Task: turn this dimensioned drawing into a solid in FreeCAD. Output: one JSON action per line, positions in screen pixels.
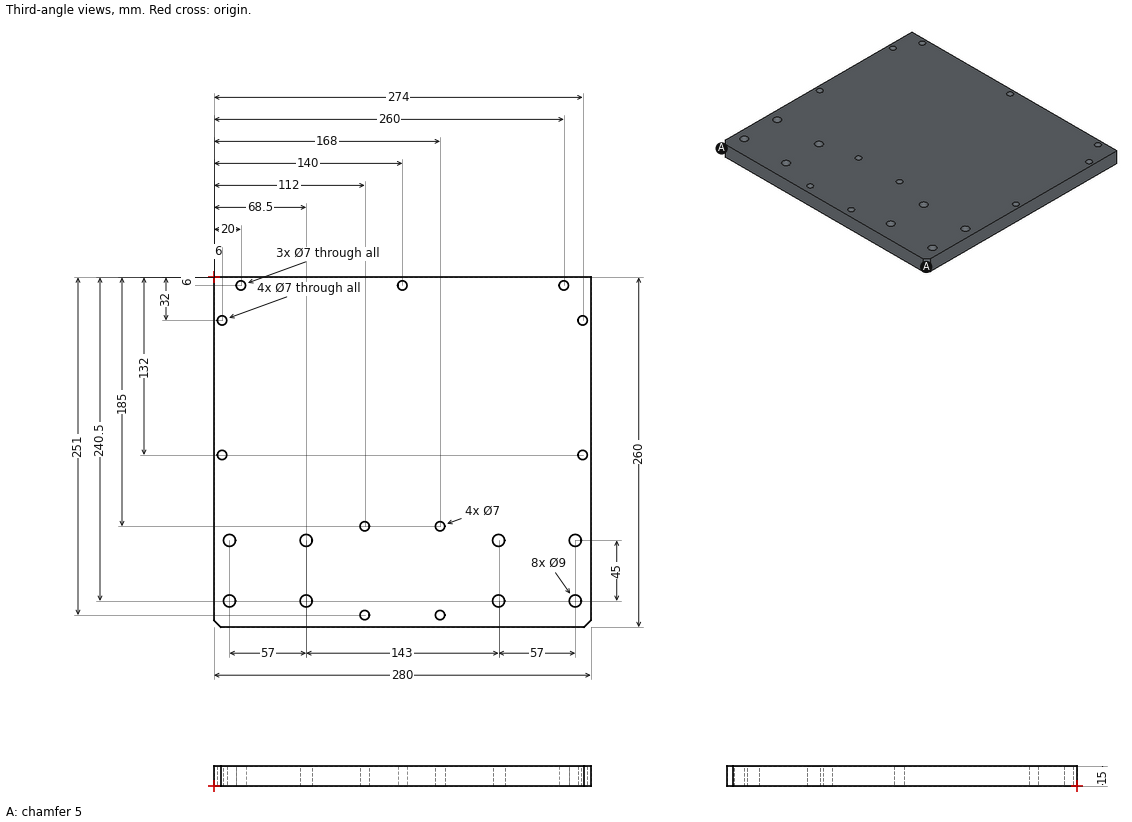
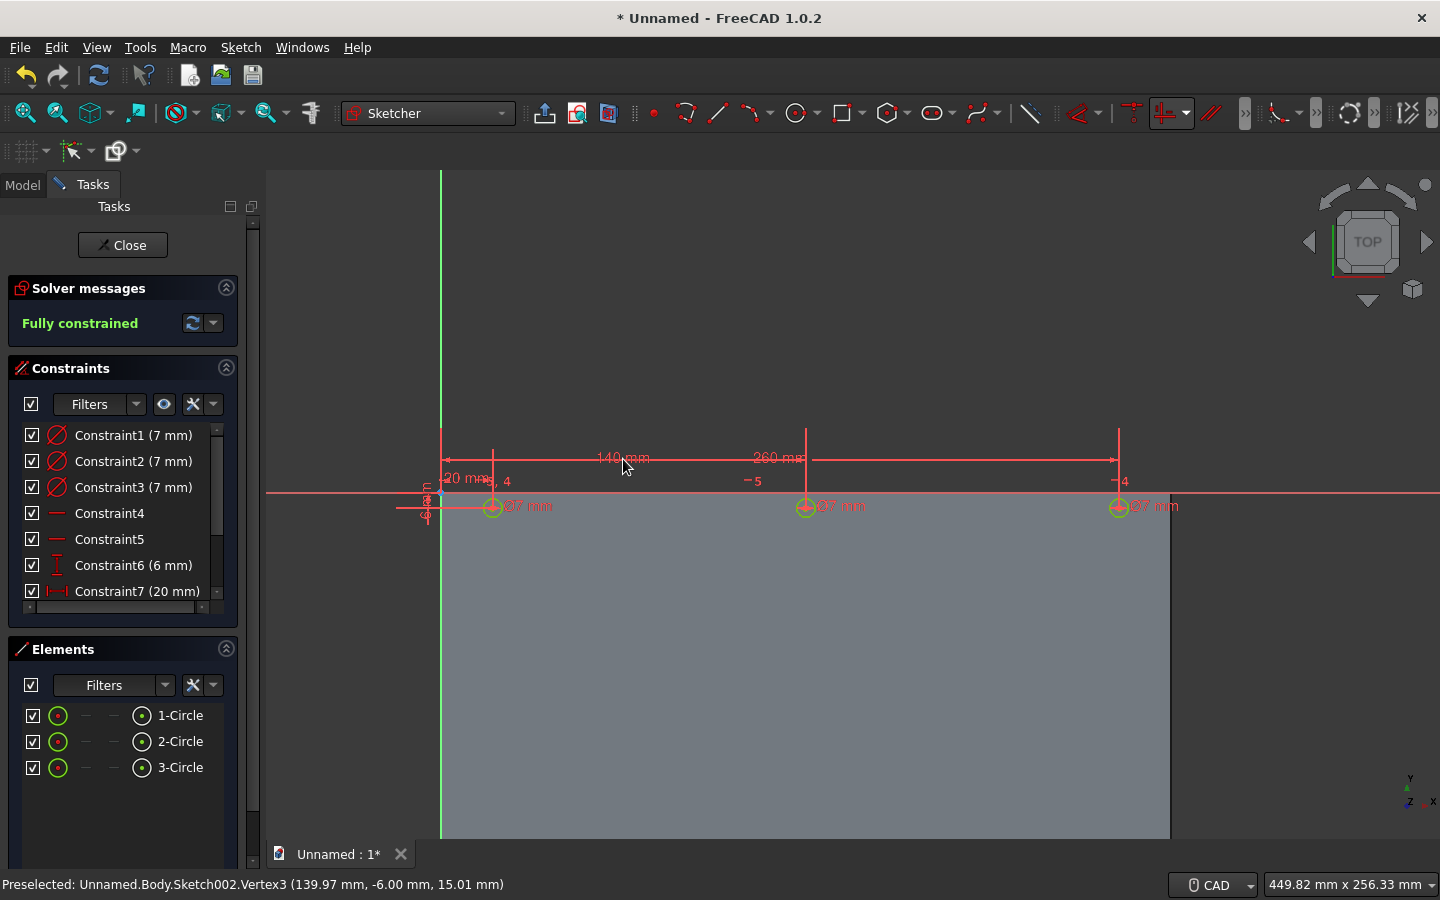
{"action": "left_click", "coordinate": [123, 245]}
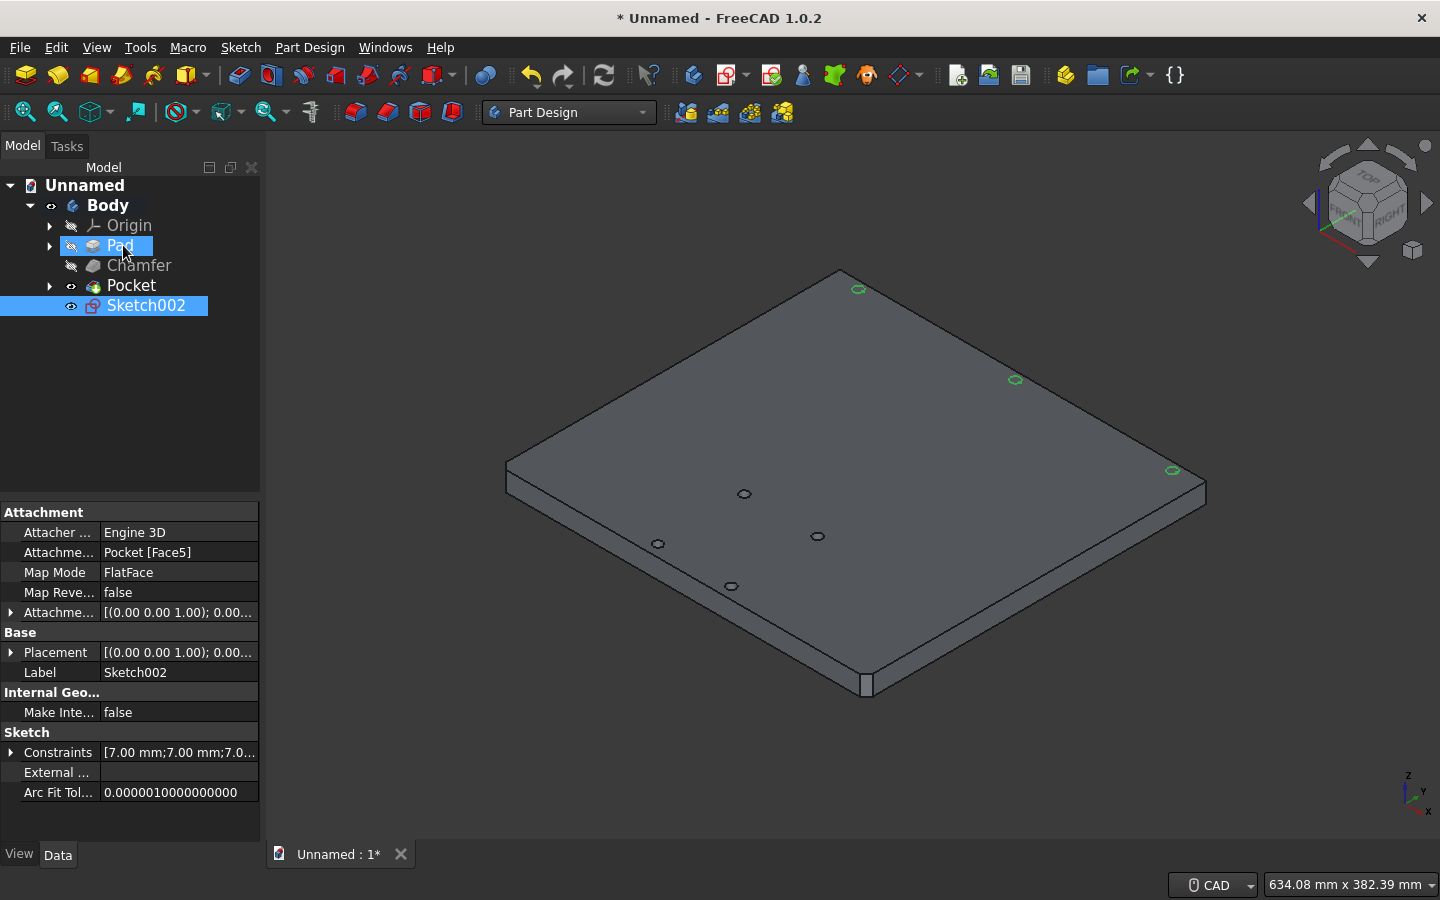
{"action": "left_click", "coordinate": [272, 76]}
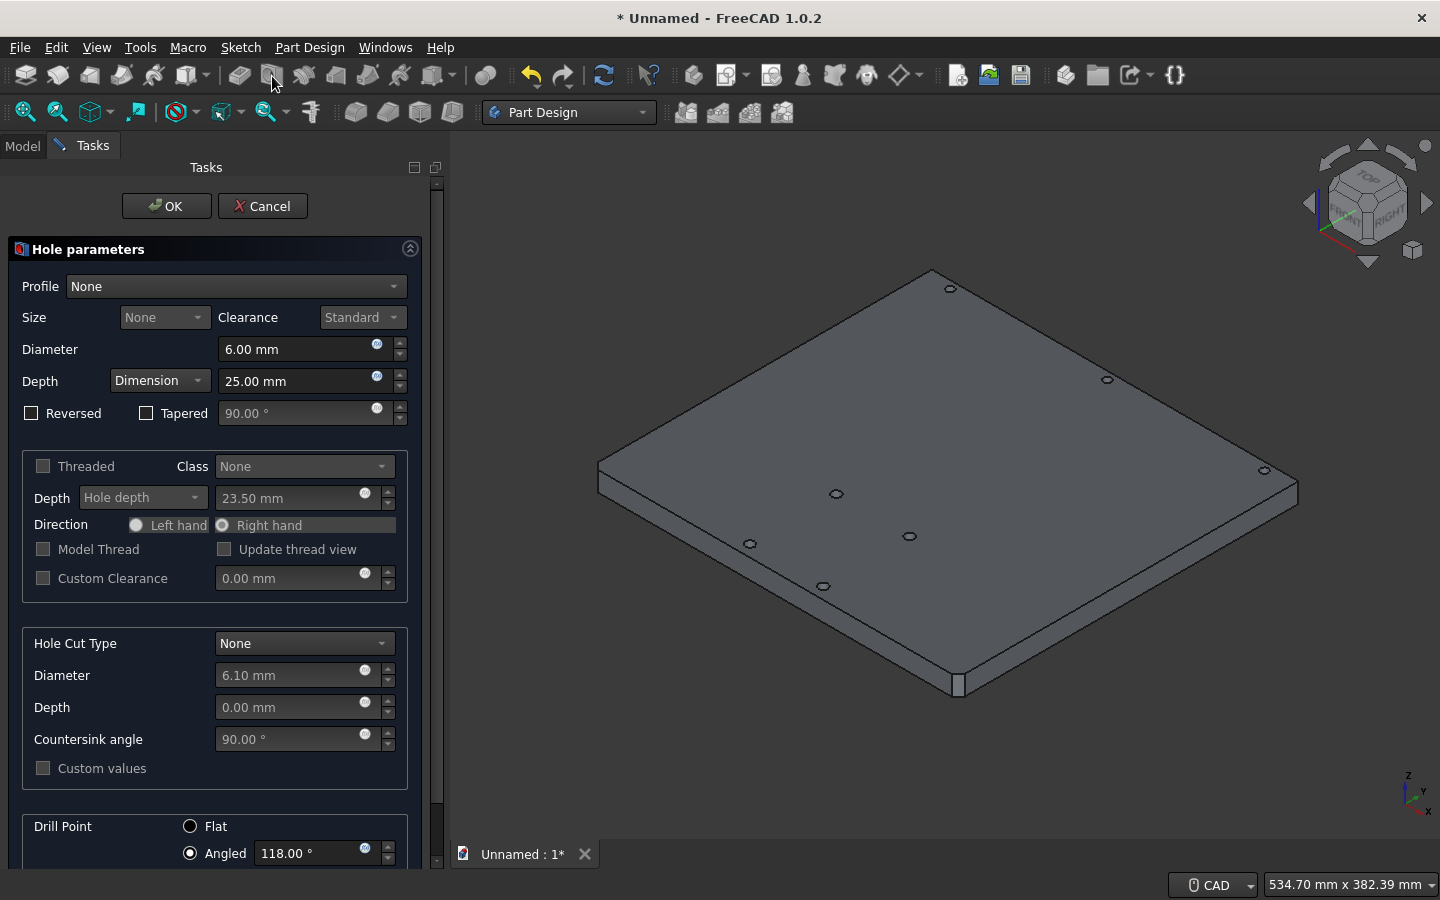
{"action": "triple_click", "coordinate": [305, 349]}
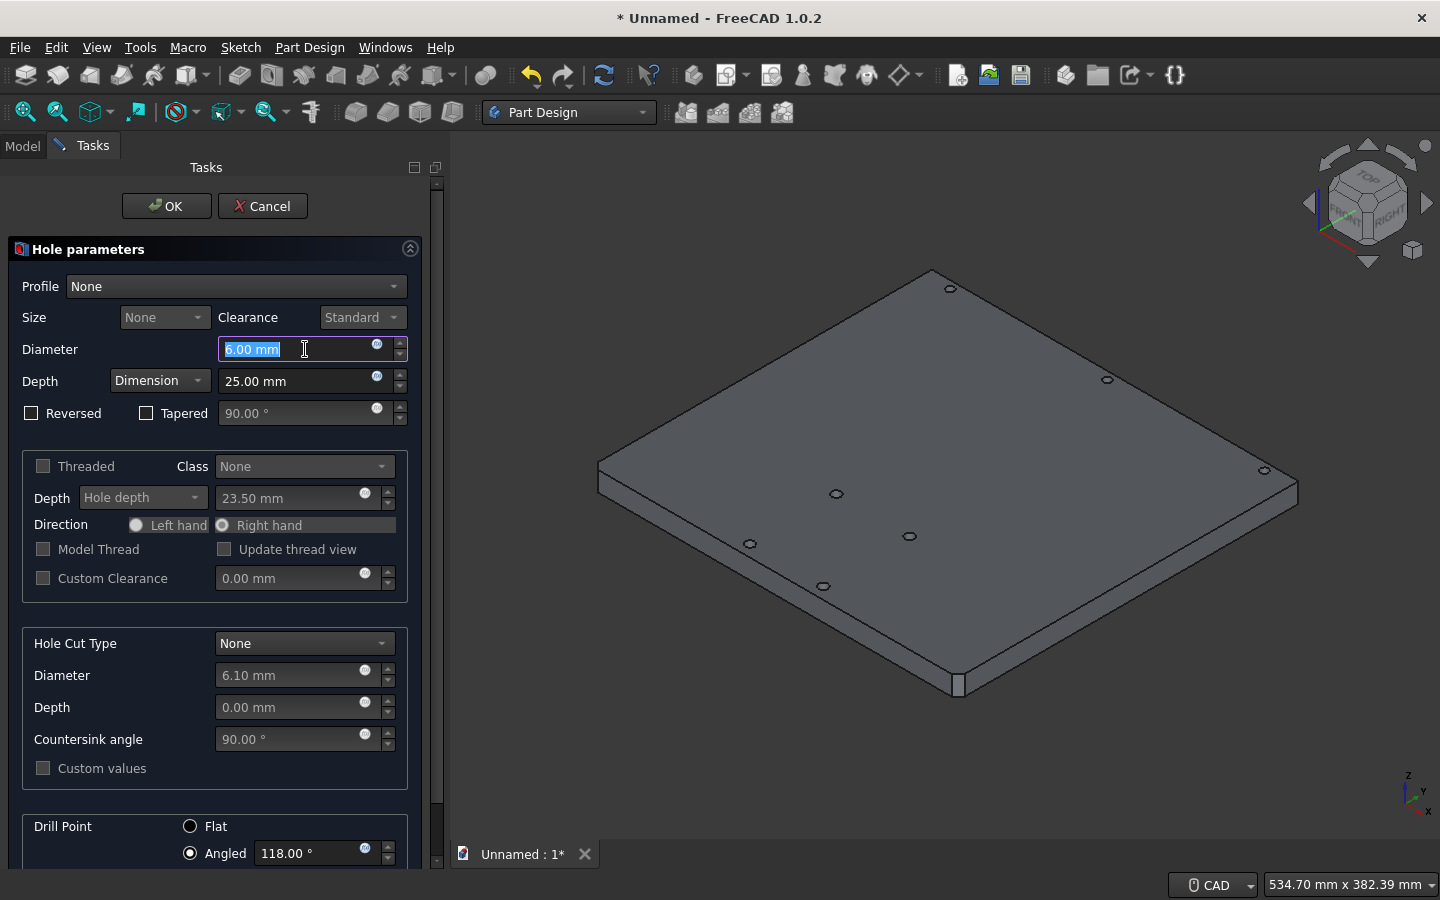
{"action": "type", "text": "7"}
{"action": "key", "text": "Tab"}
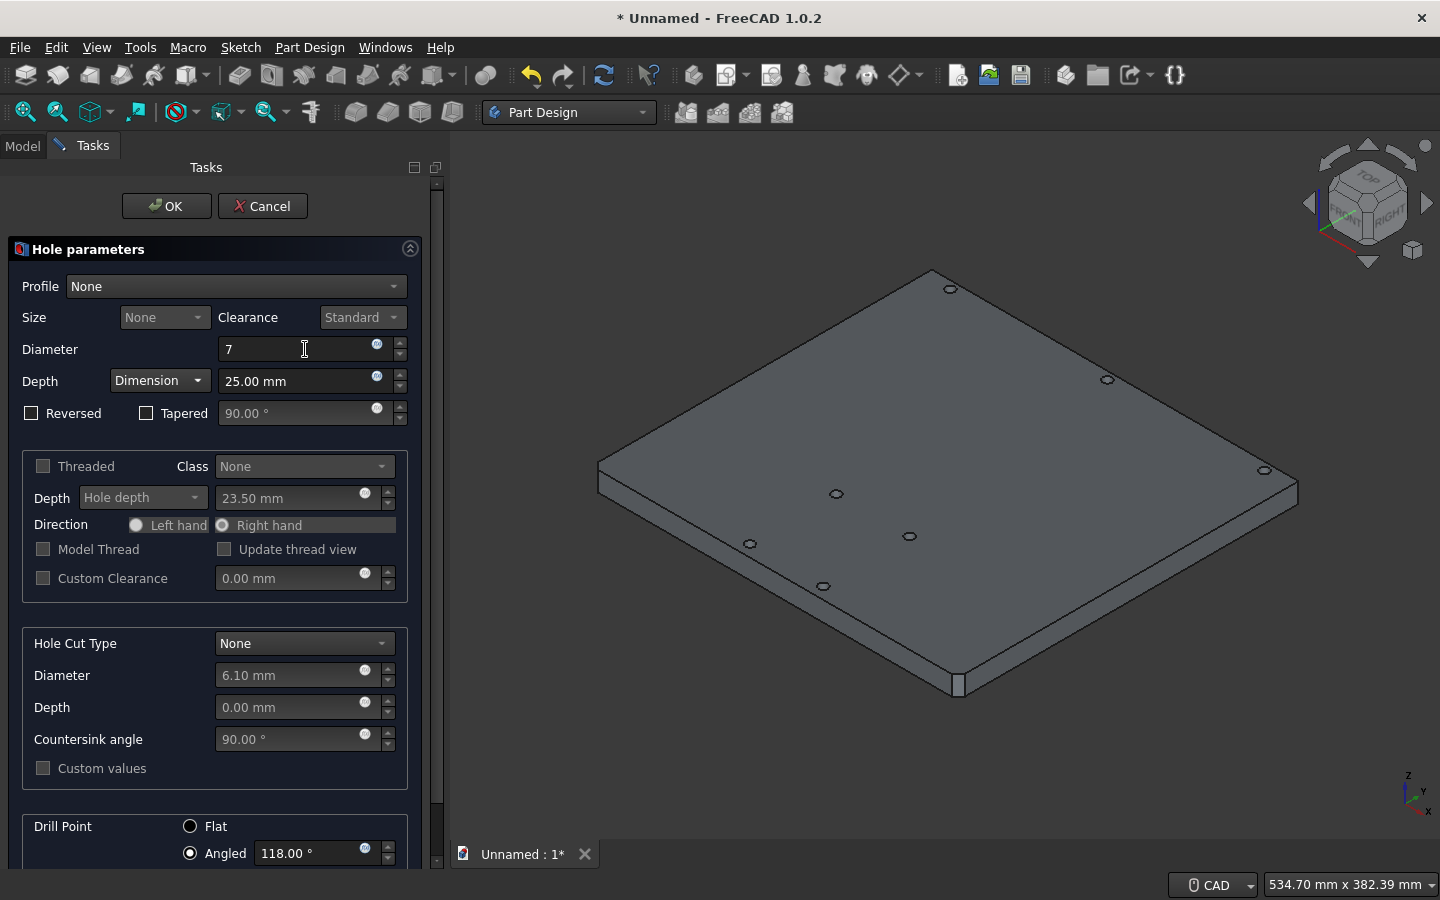
{"action": "left_click", "coordinate": [161, 380]}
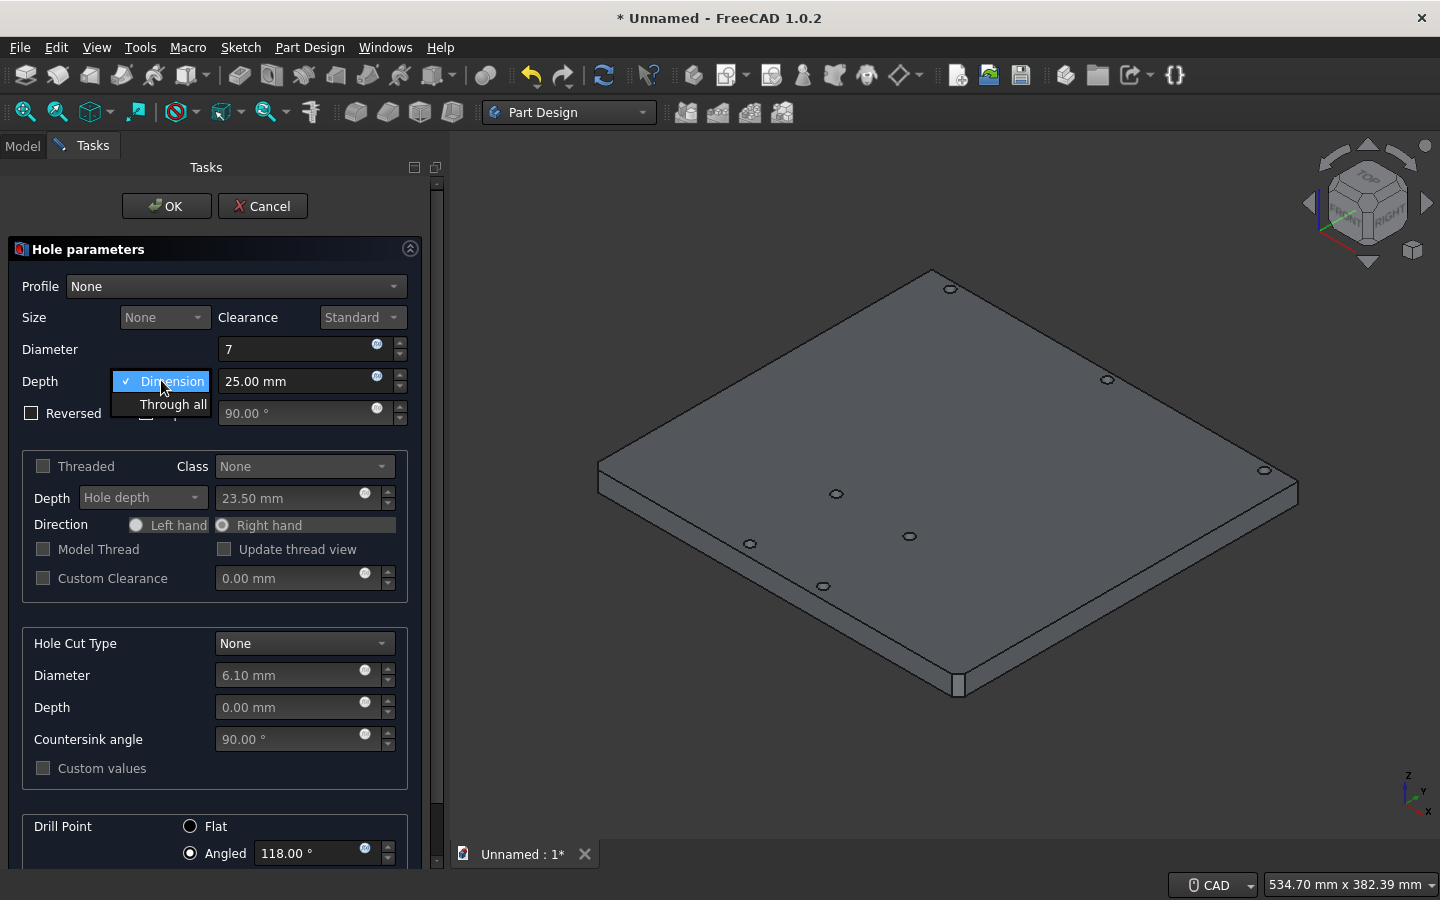
{"action": "left_click", "coordinate": [160, 404]}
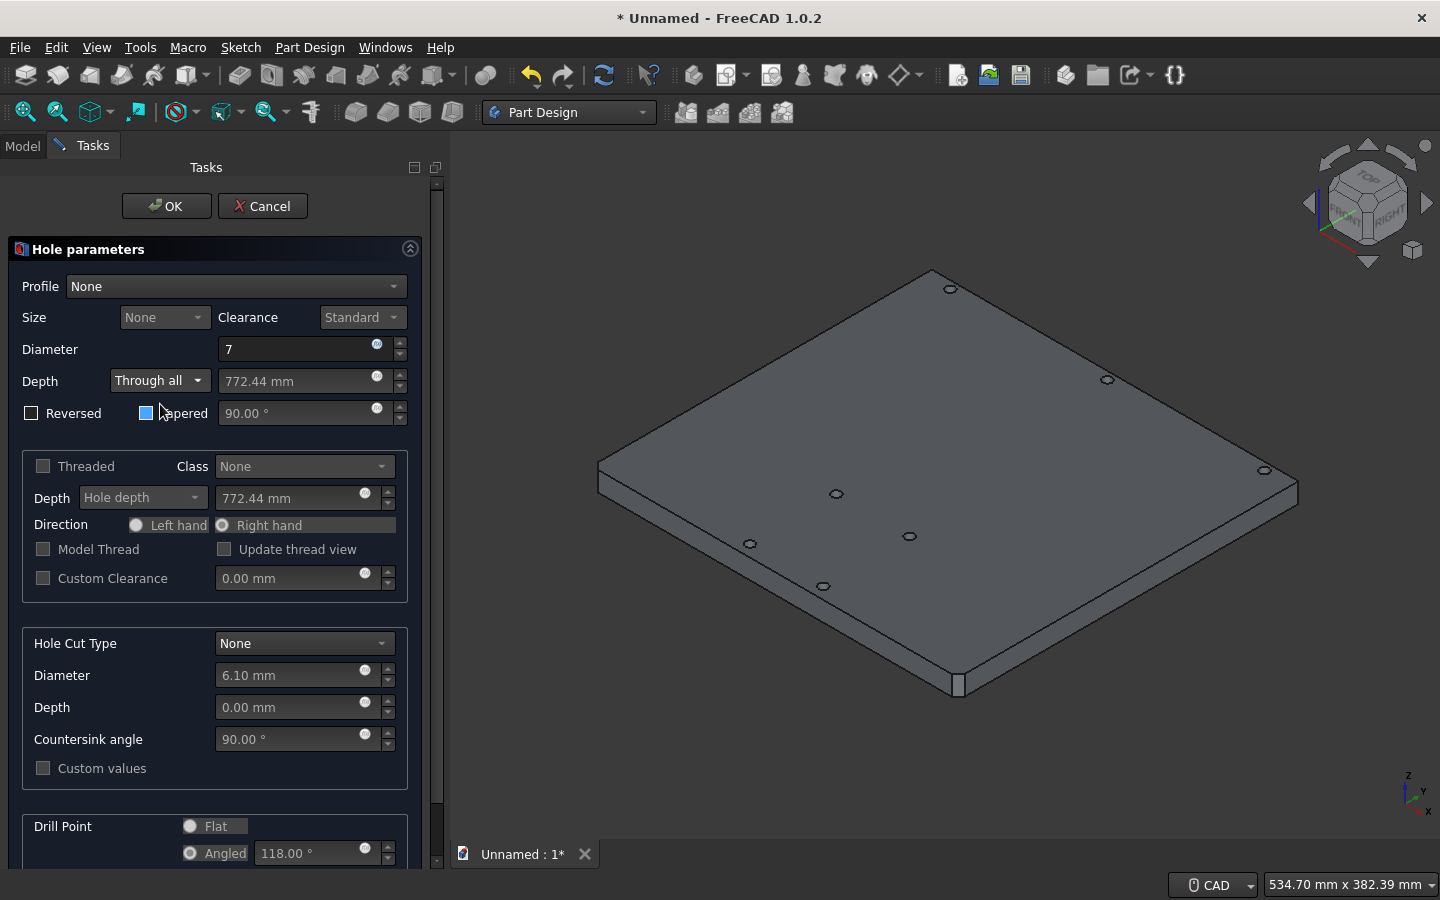
{"action": "left_click", "coordinate": [167, 206]}